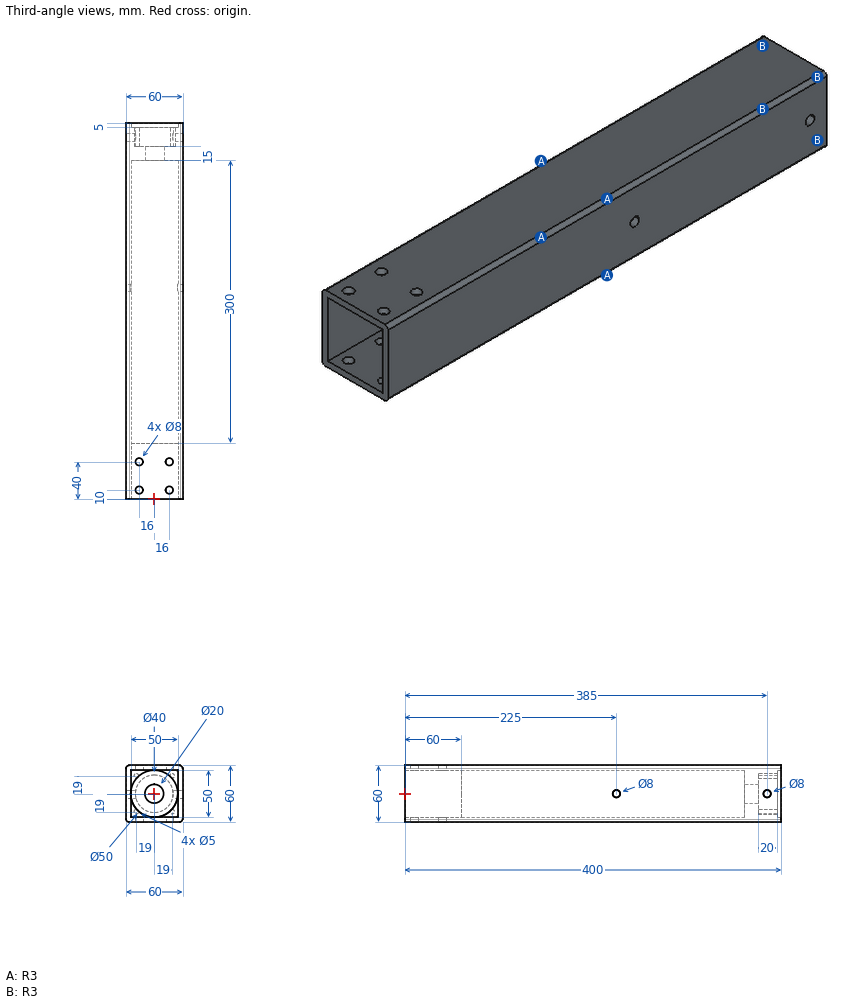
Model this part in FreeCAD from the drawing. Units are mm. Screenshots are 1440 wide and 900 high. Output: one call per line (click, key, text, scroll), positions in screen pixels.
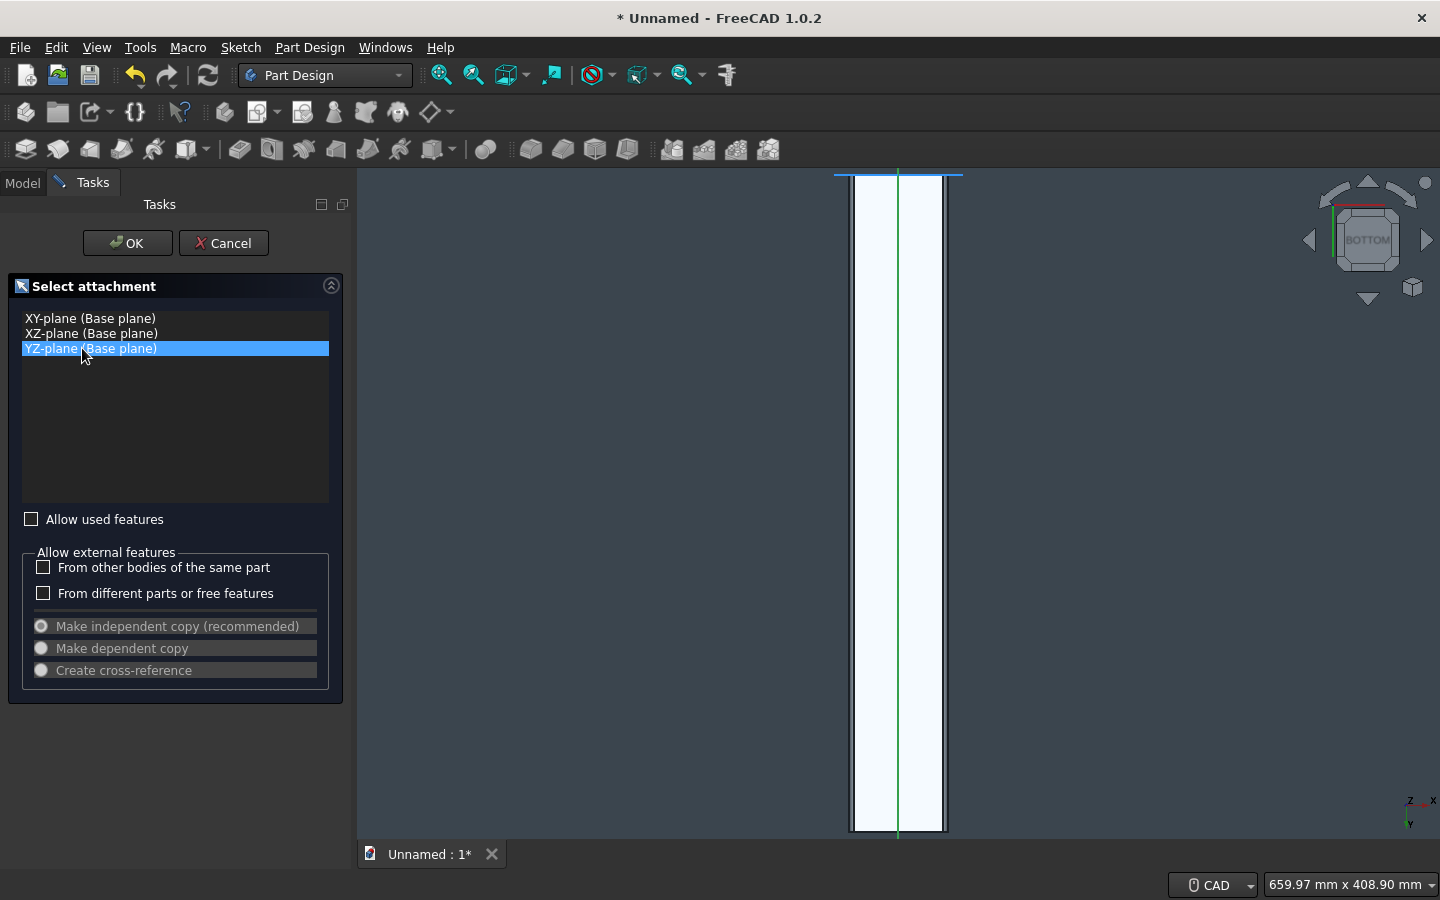
click(128, 243)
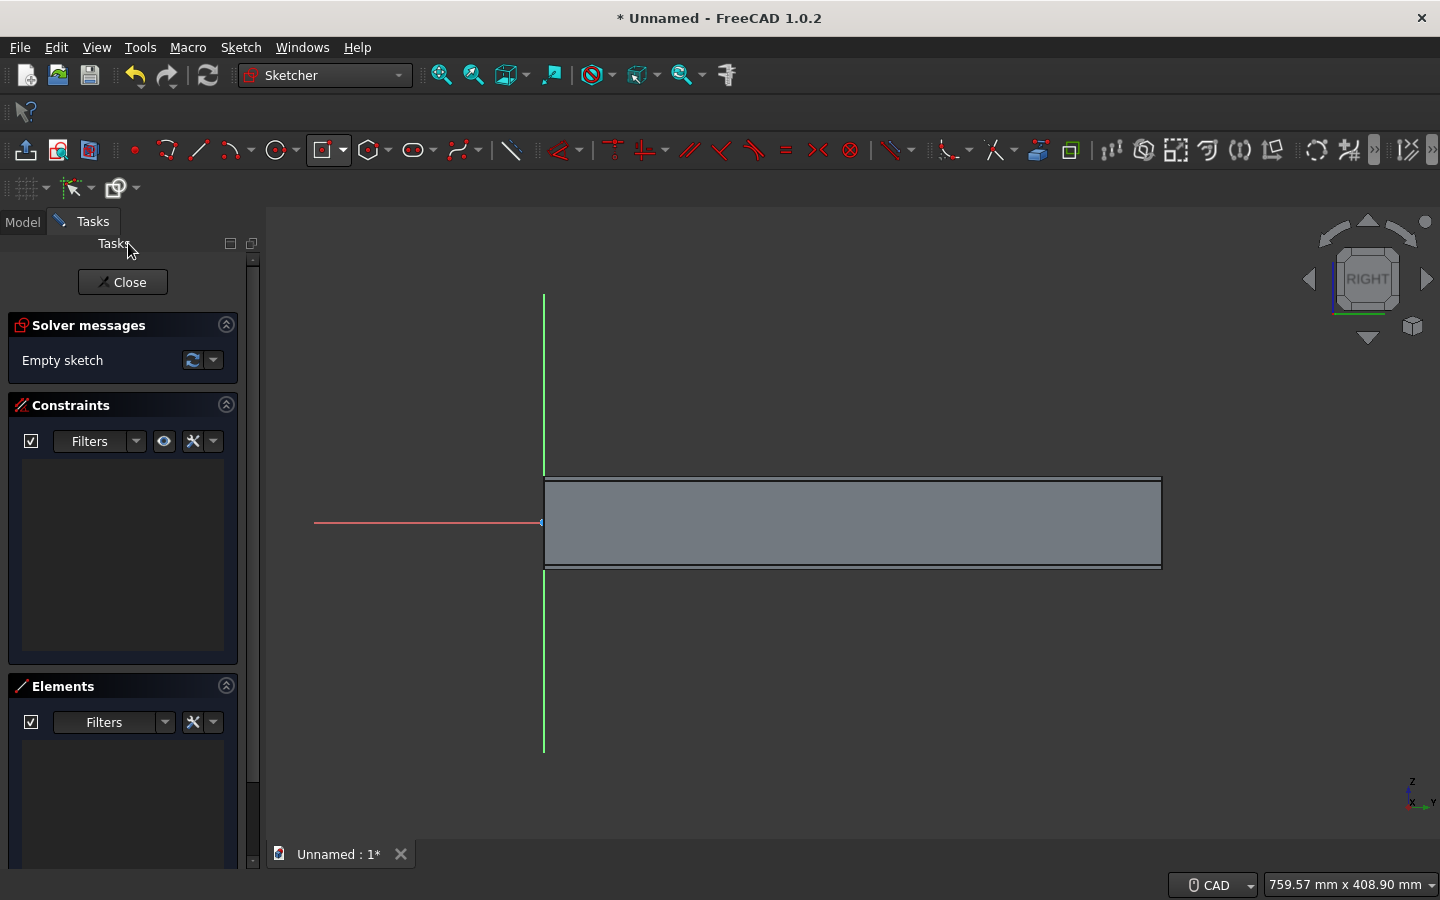
click(90, 150)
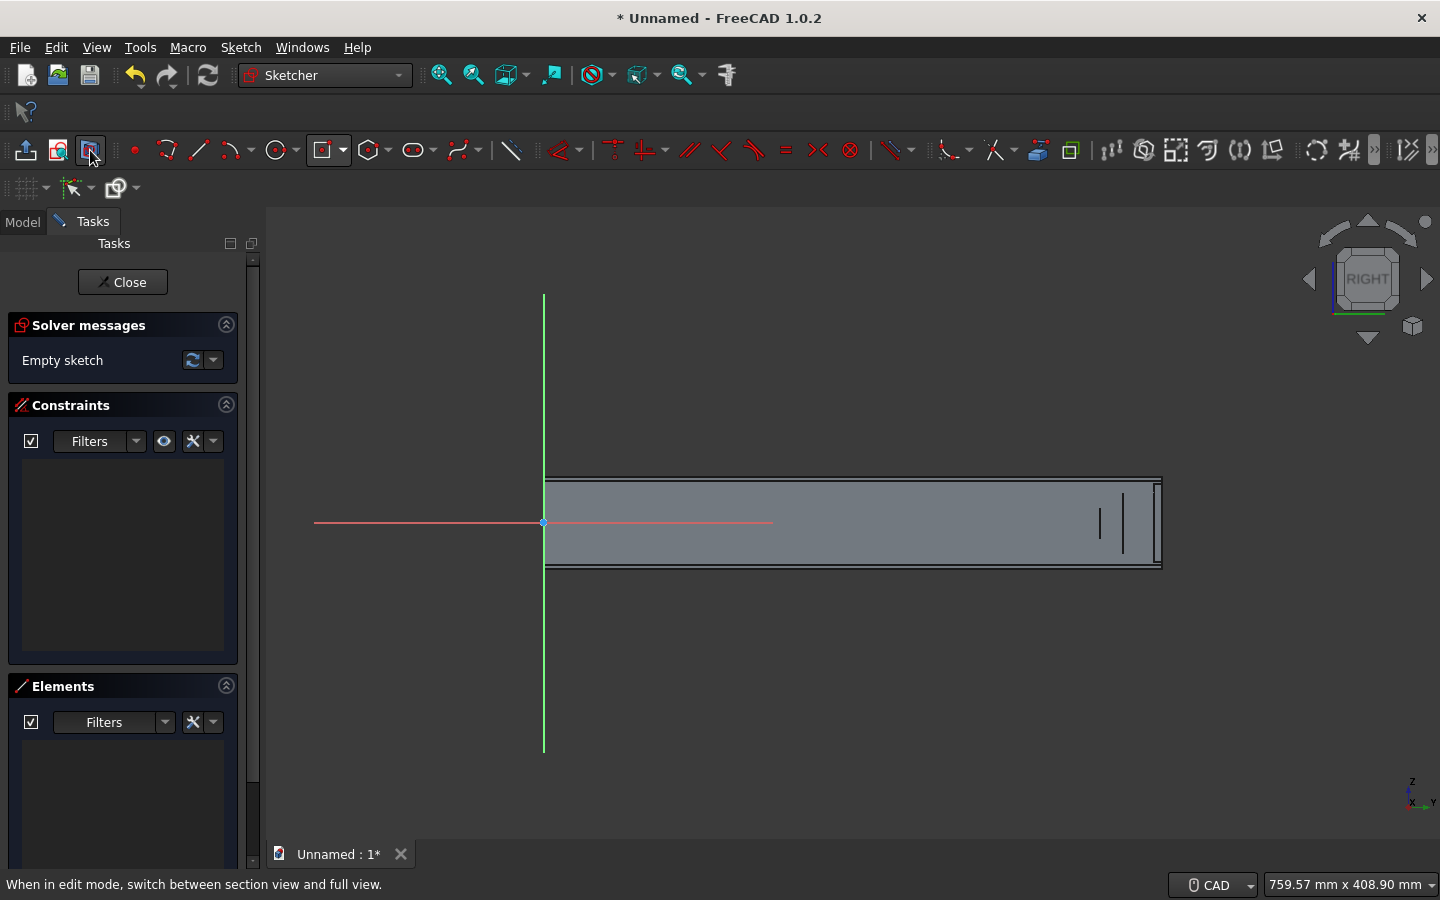
scroll(1158, 523, up, 15)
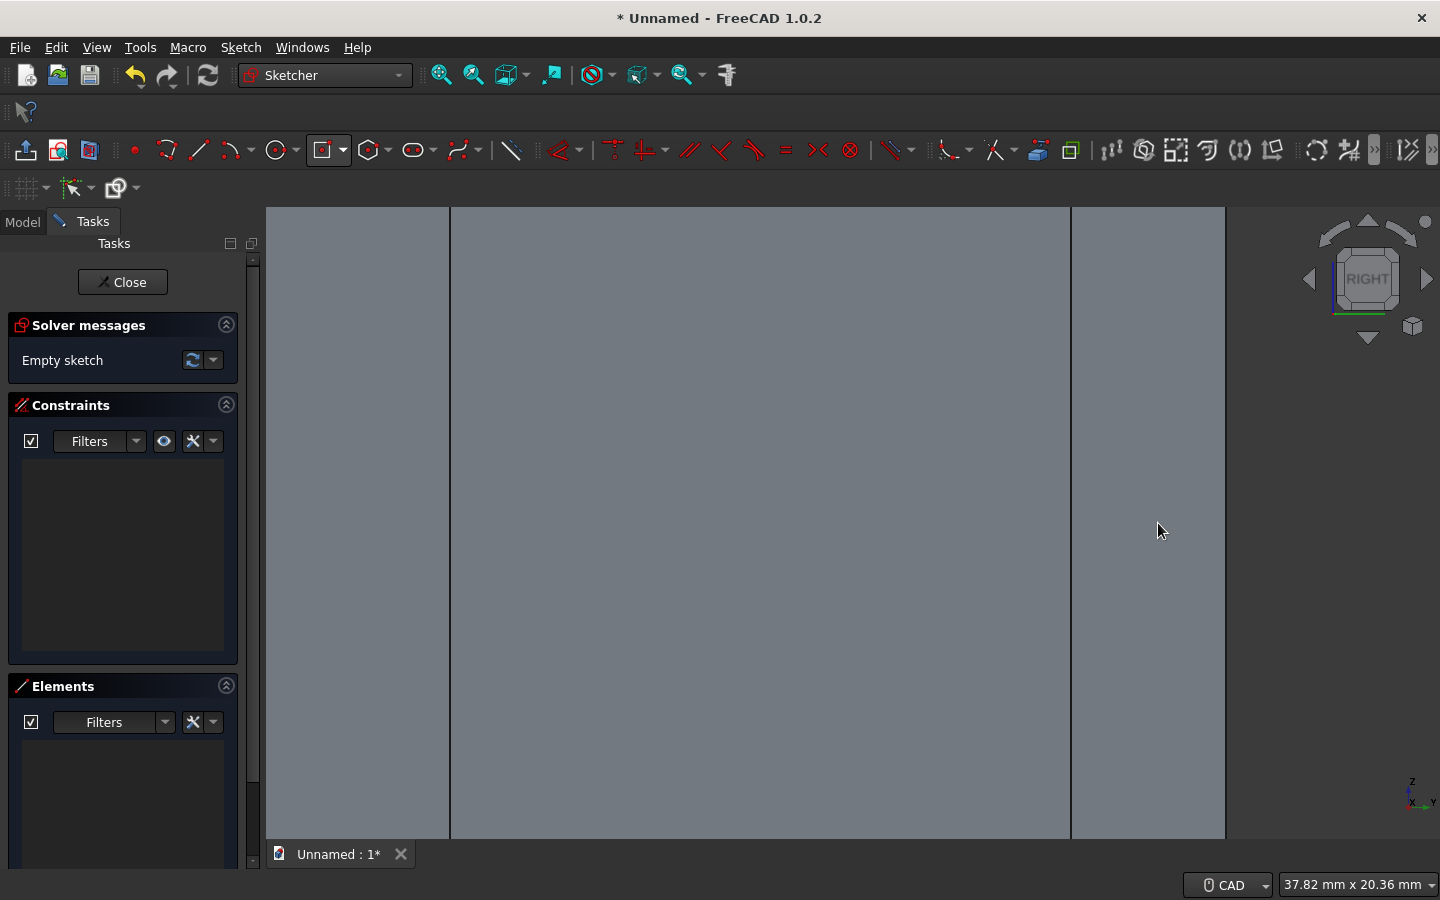
scroll(712, 494, up, 2)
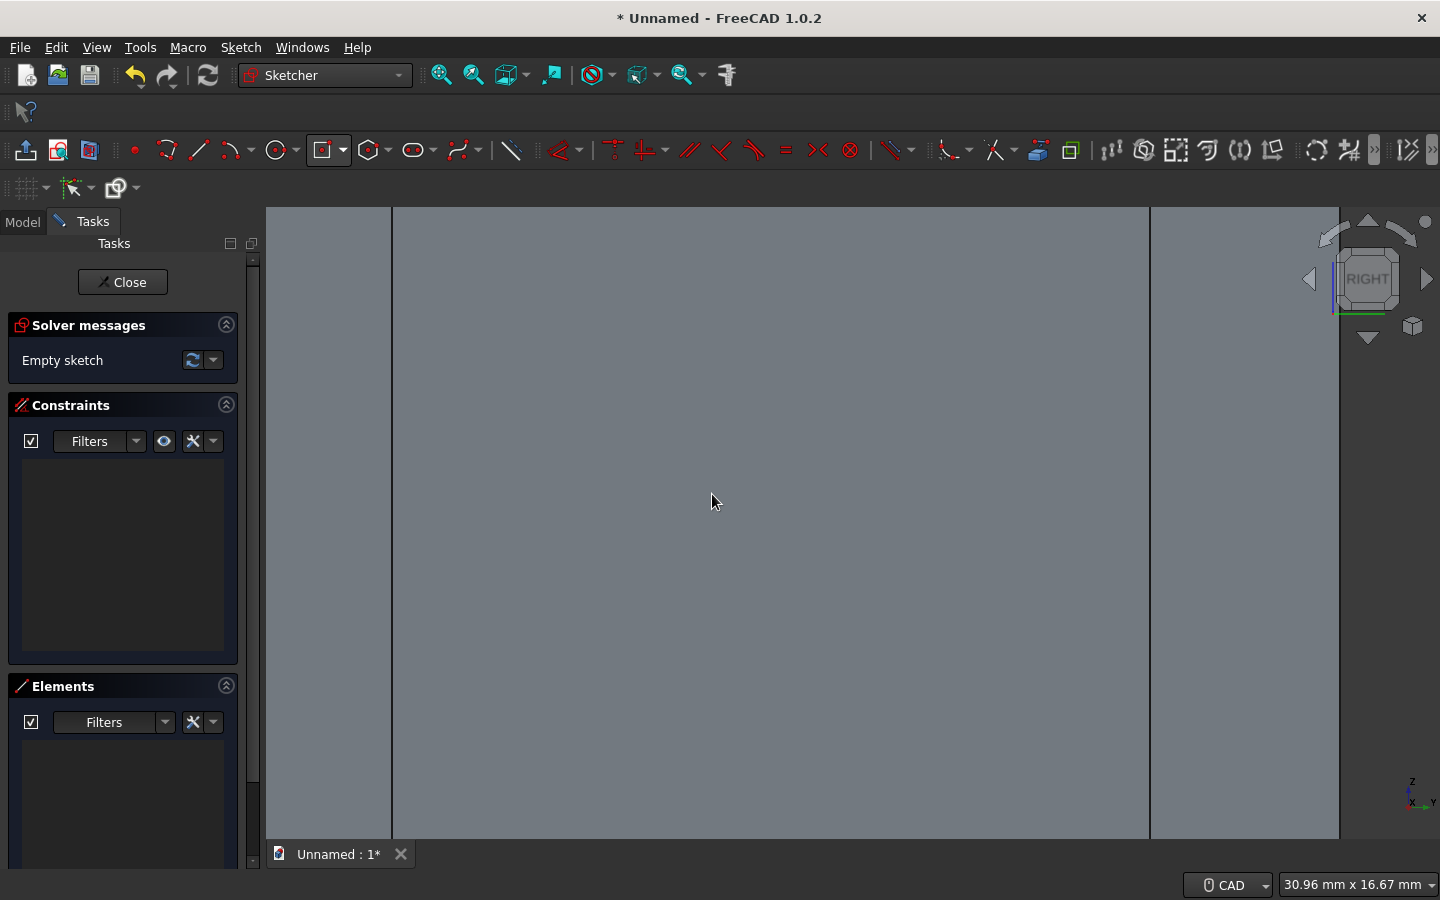
click(276, 150)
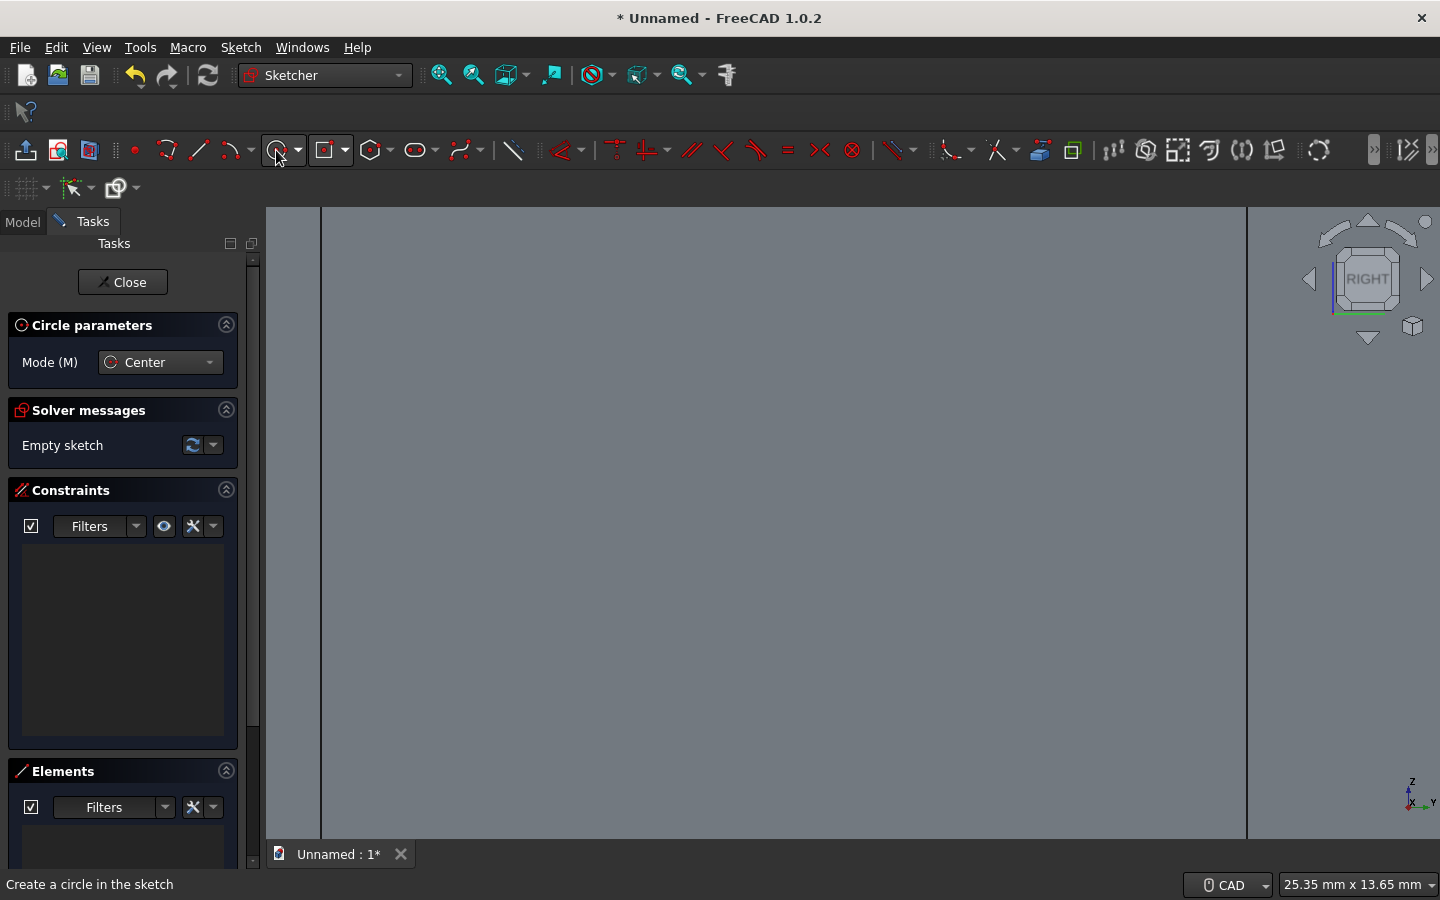
click(784, 523)
move(915, 392)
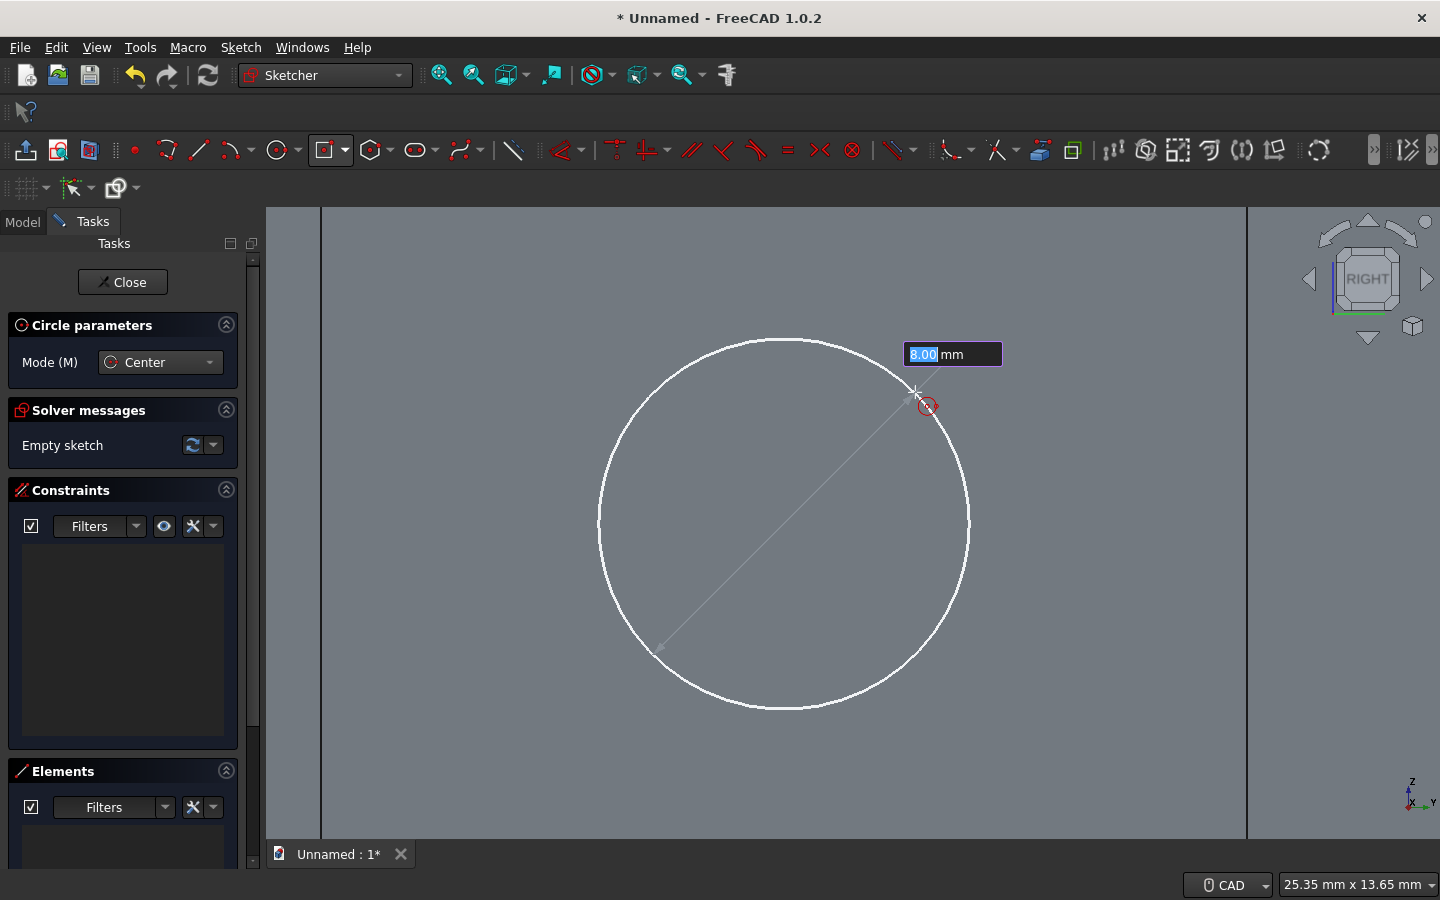
text(8)
key(Return)
key(Escape)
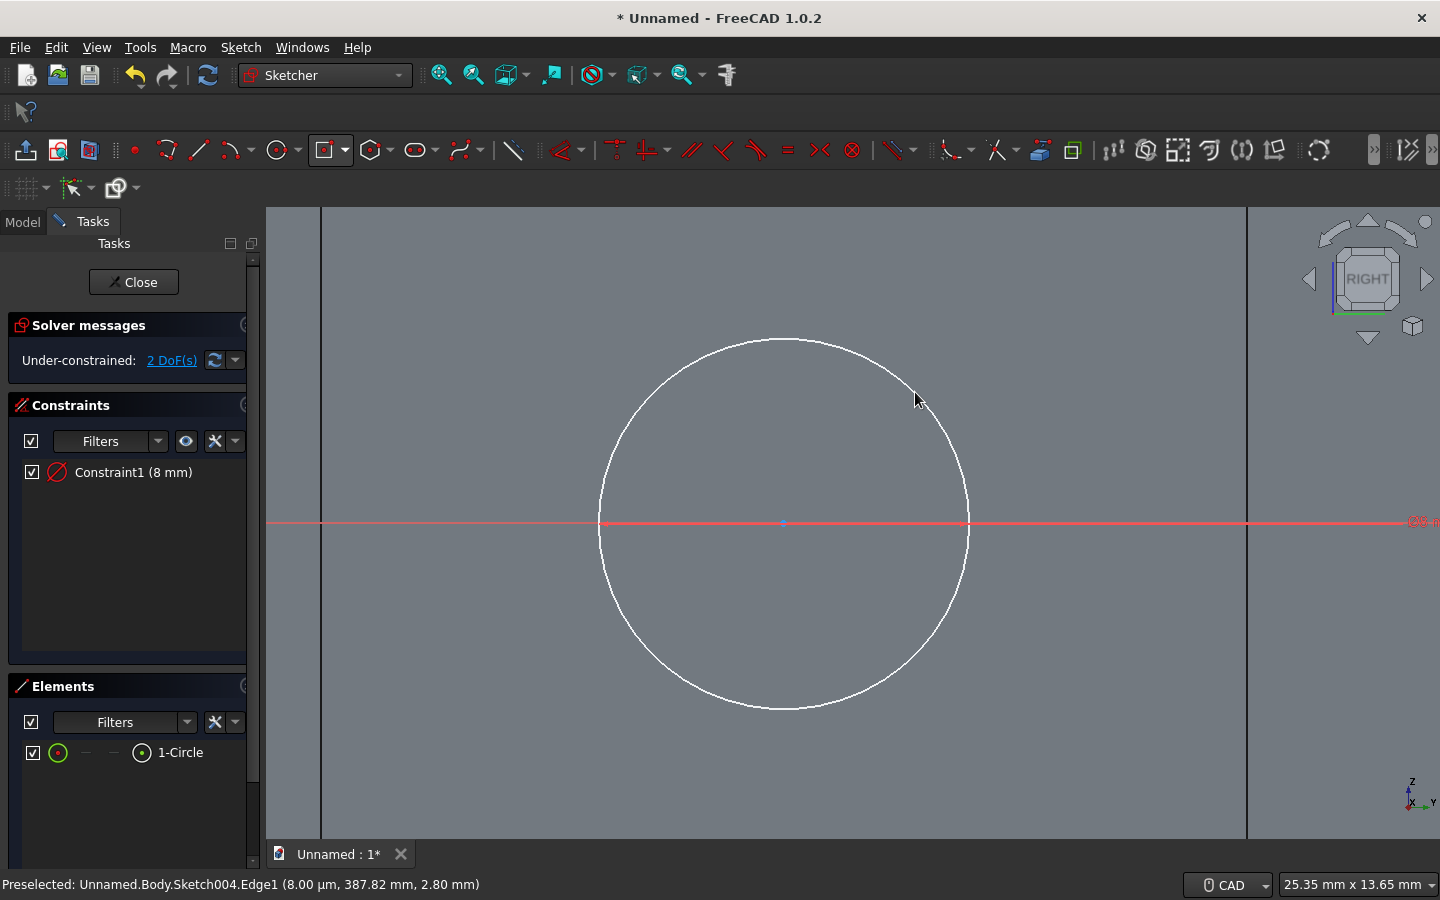
click(784, 524)